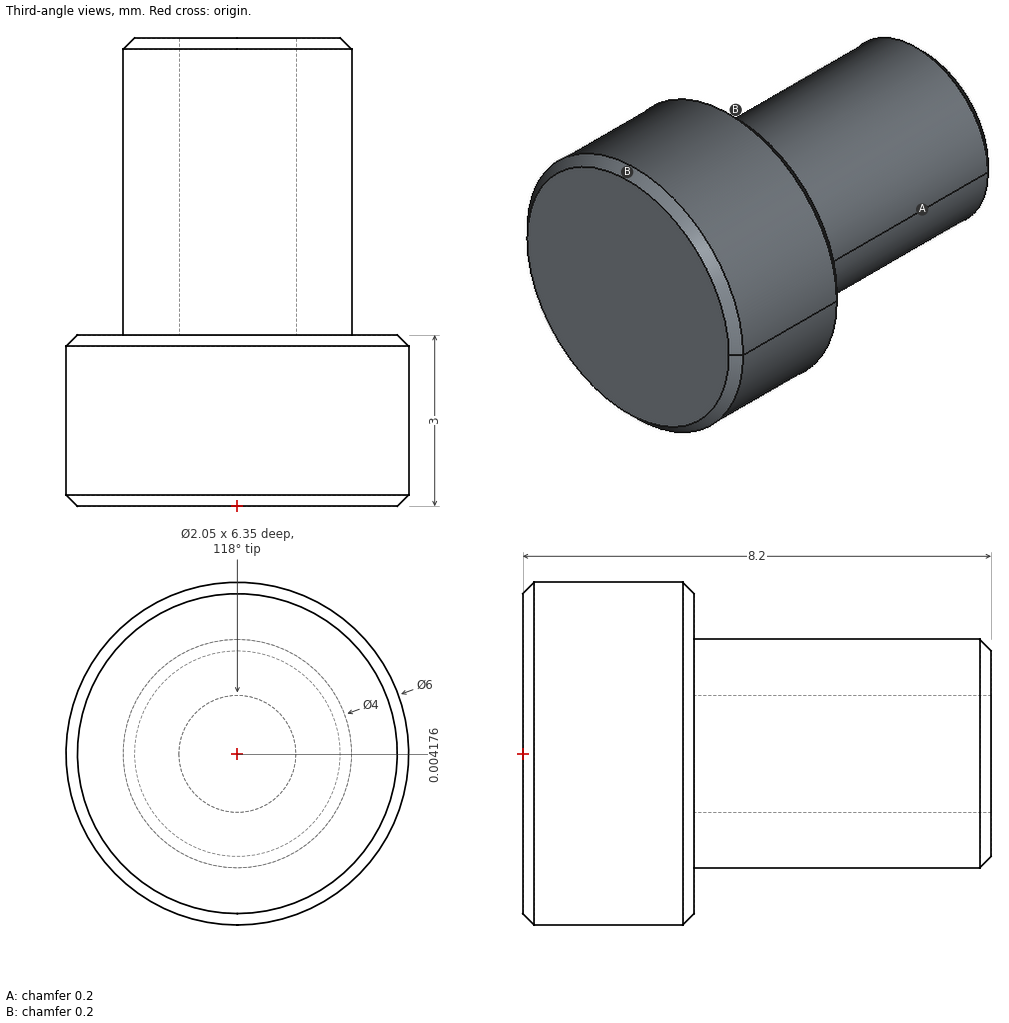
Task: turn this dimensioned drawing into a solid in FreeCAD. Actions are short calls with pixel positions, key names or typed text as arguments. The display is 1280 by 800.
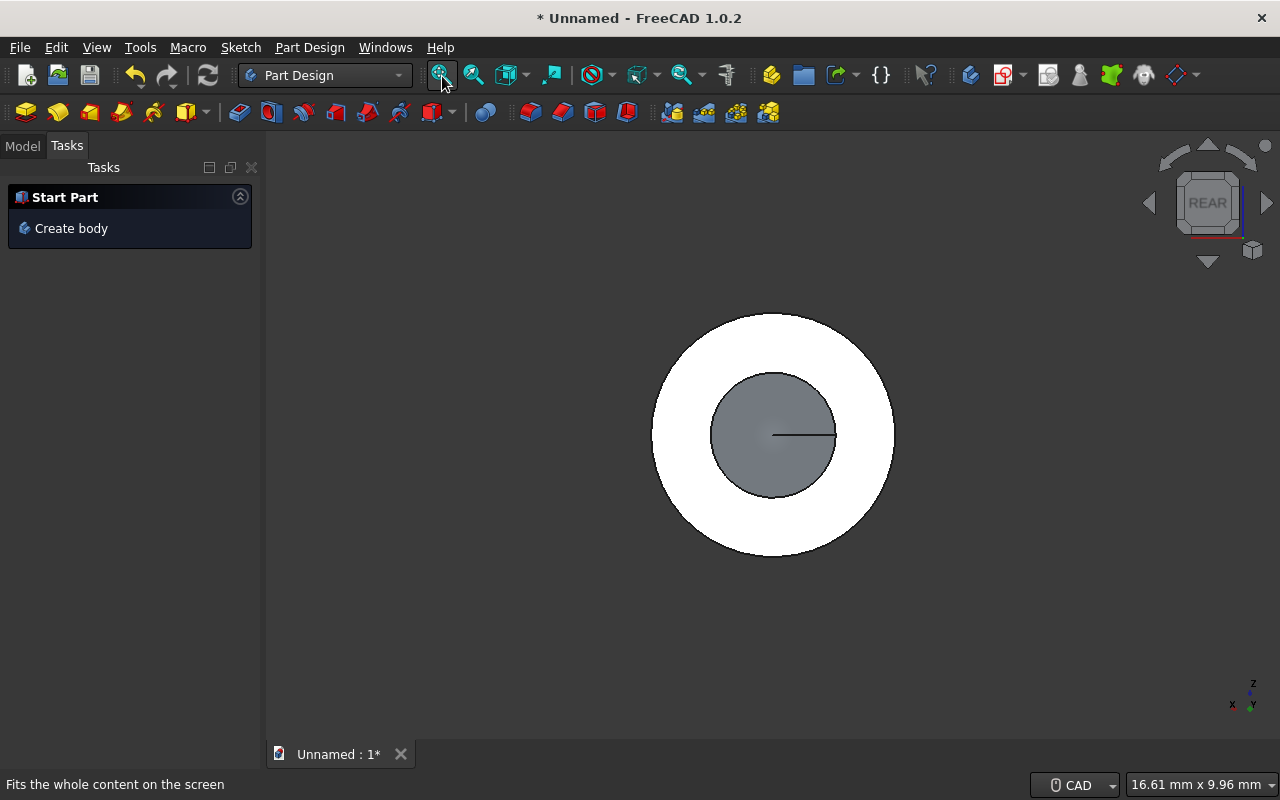
click(1004, 76)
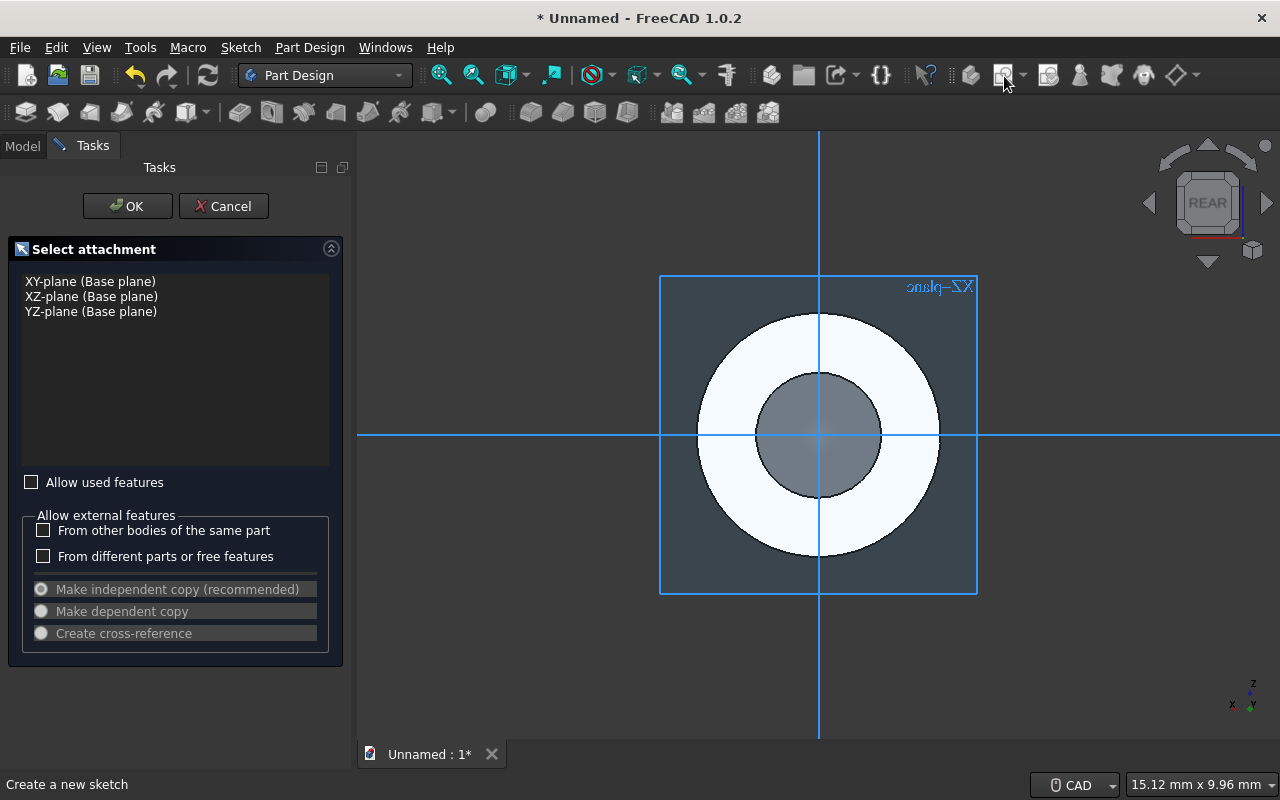
click(82, 296)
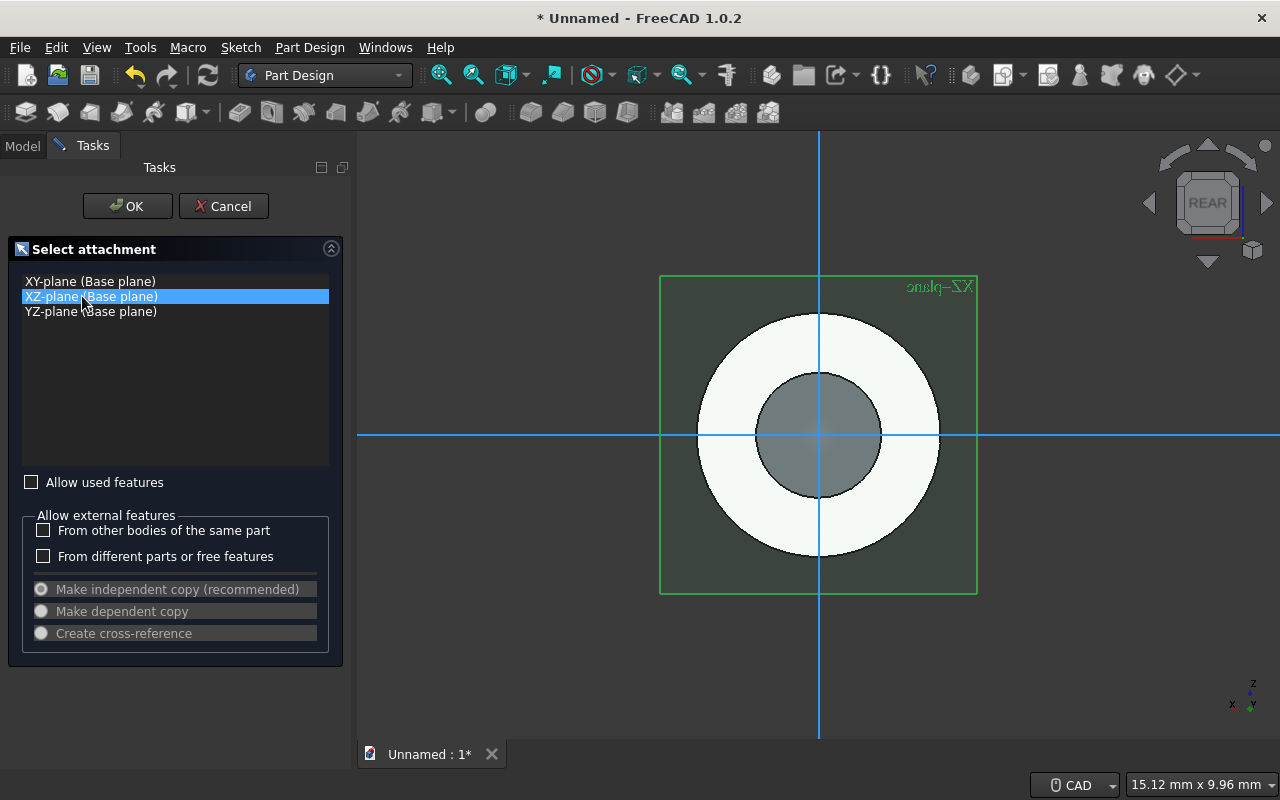
click(128, 206)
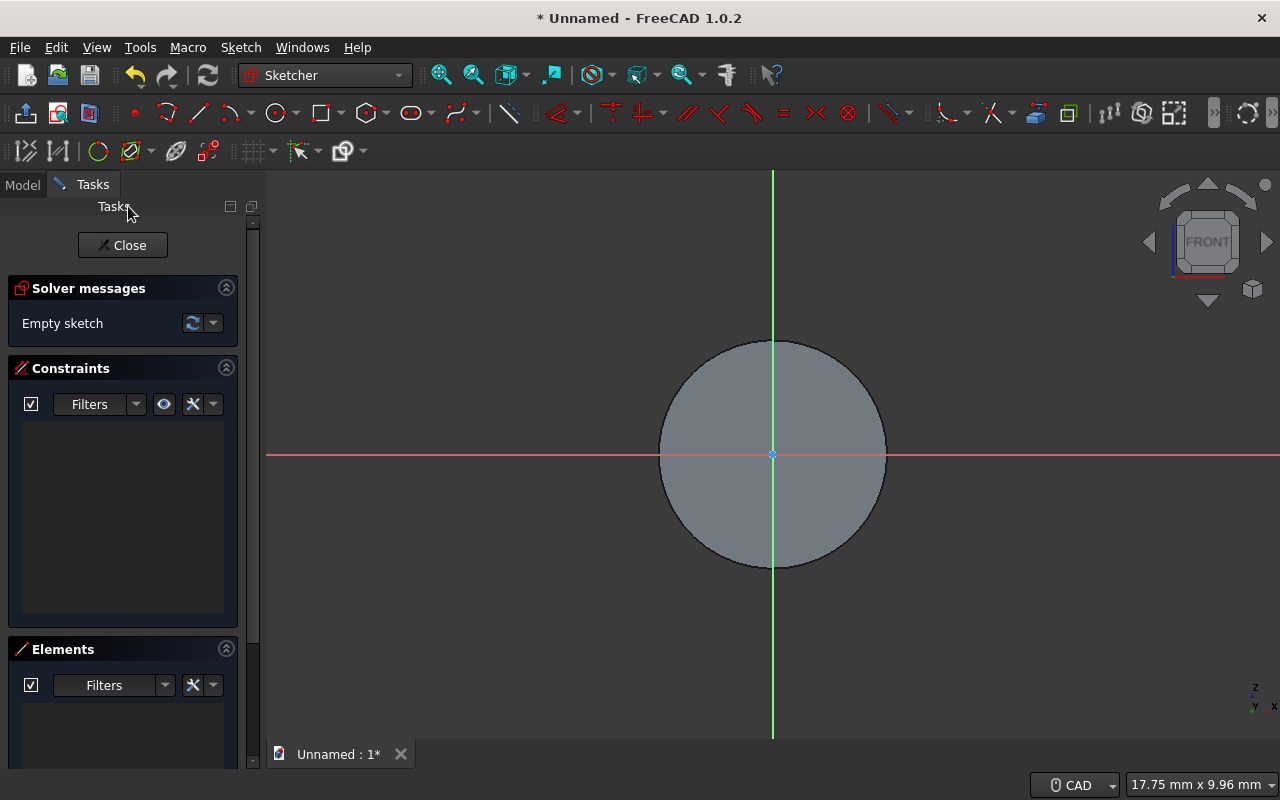
click(276, 114)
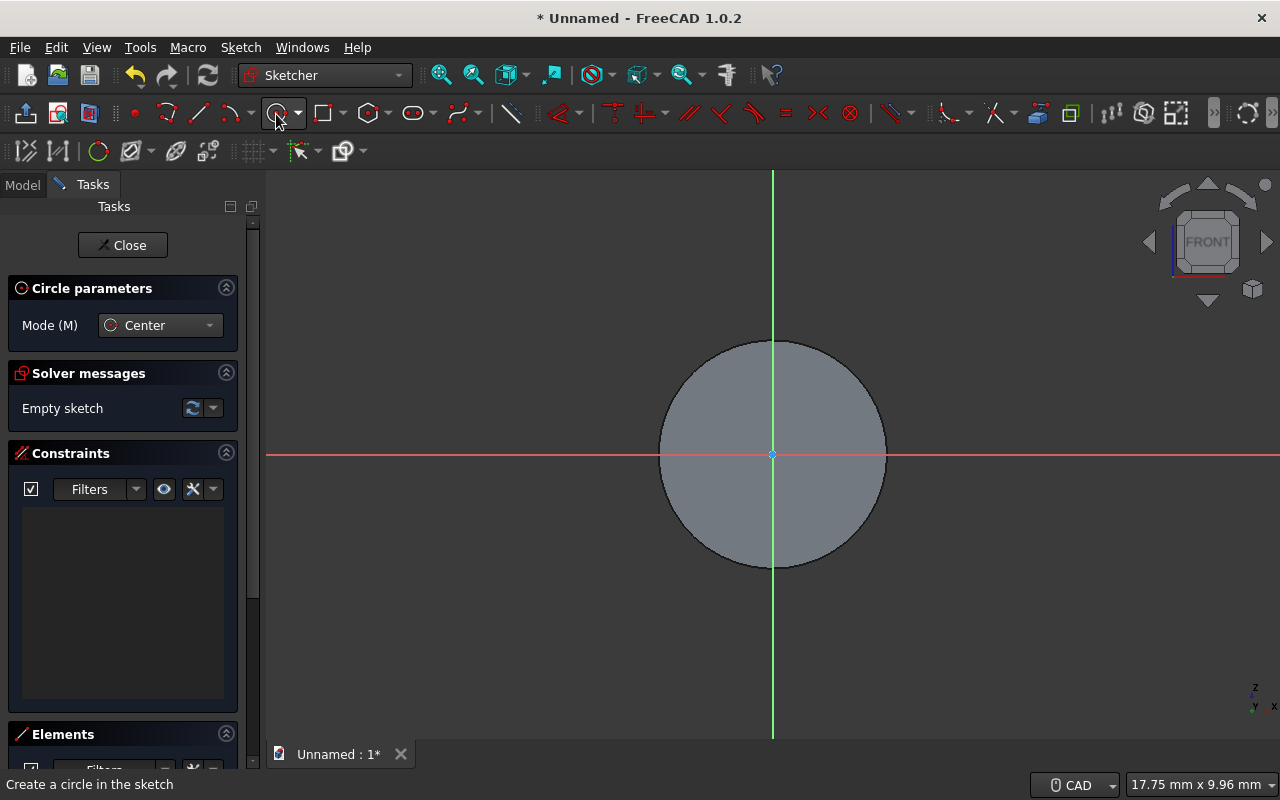
click(773, 455)
click(894, 333)
key(Escape)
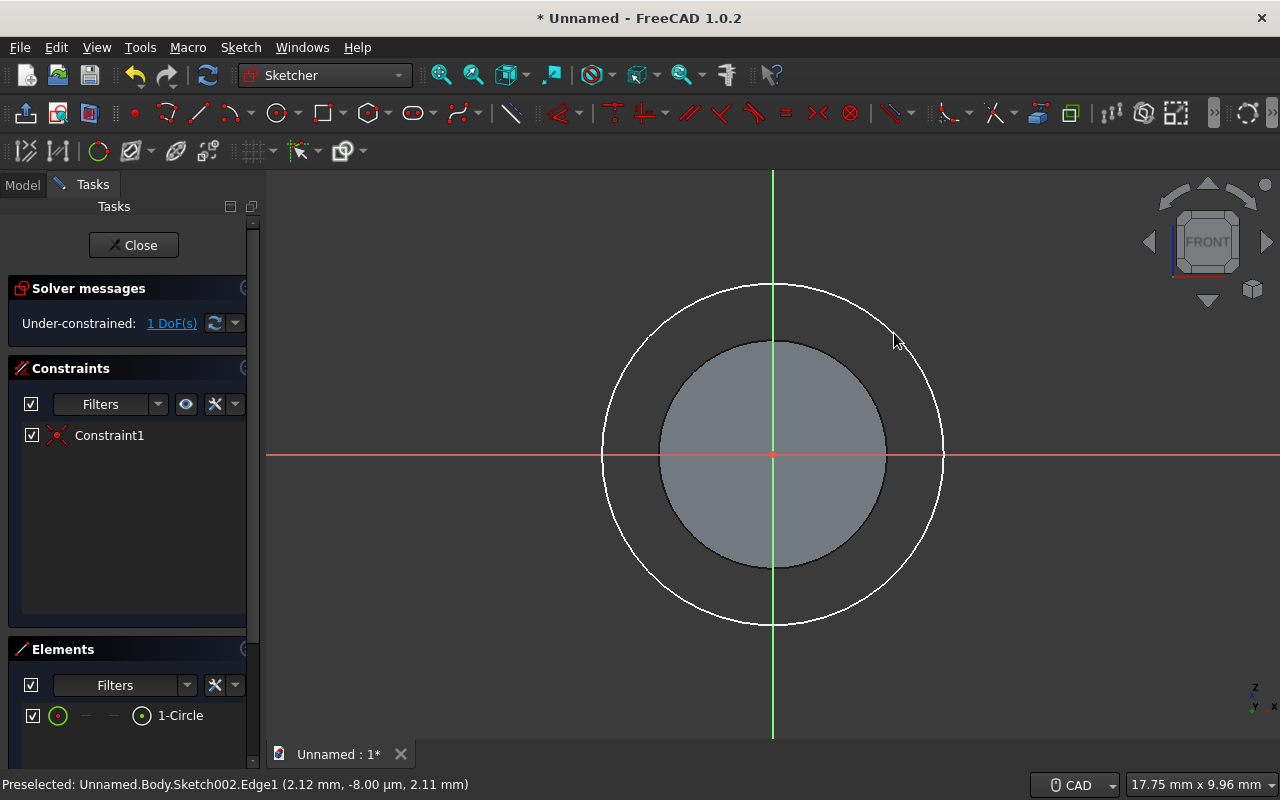
click(558, 114)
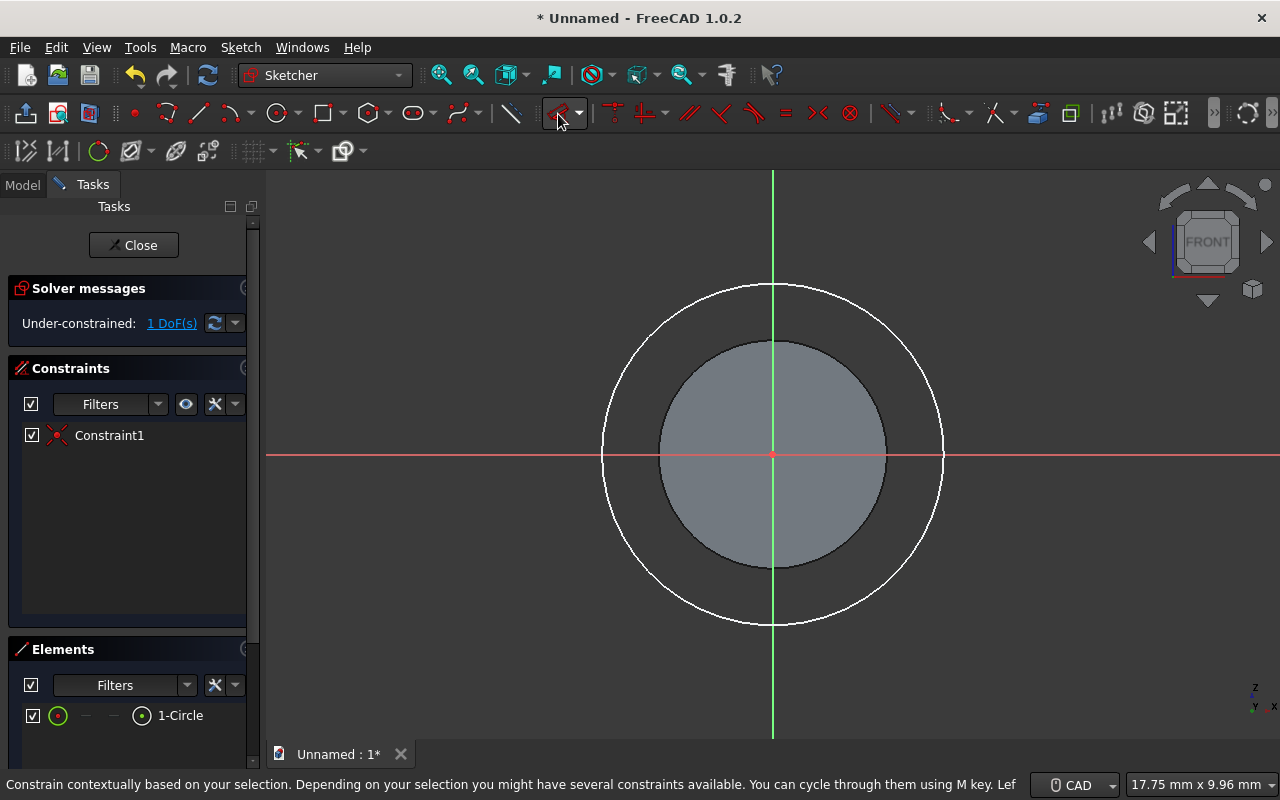
click(893, 333)
click(916, 310)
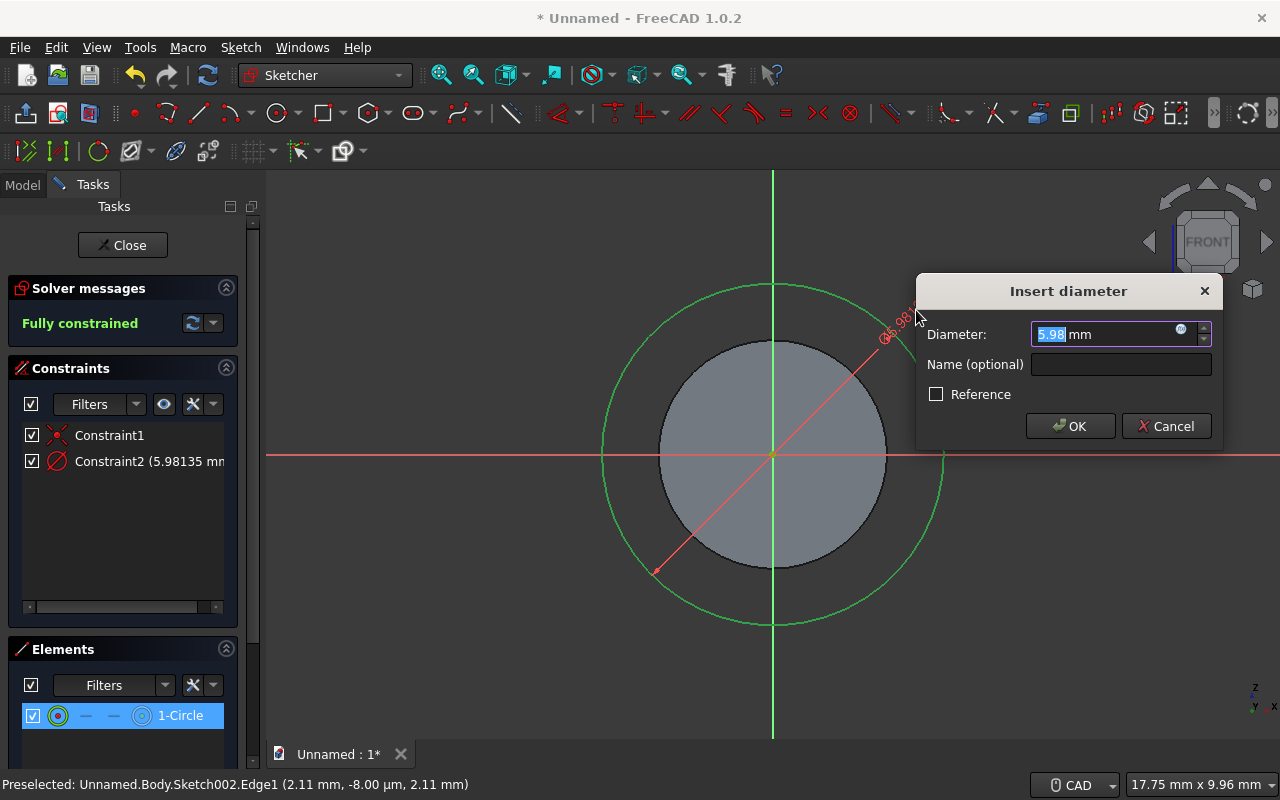
text(6)
key(Return)
key(Escape)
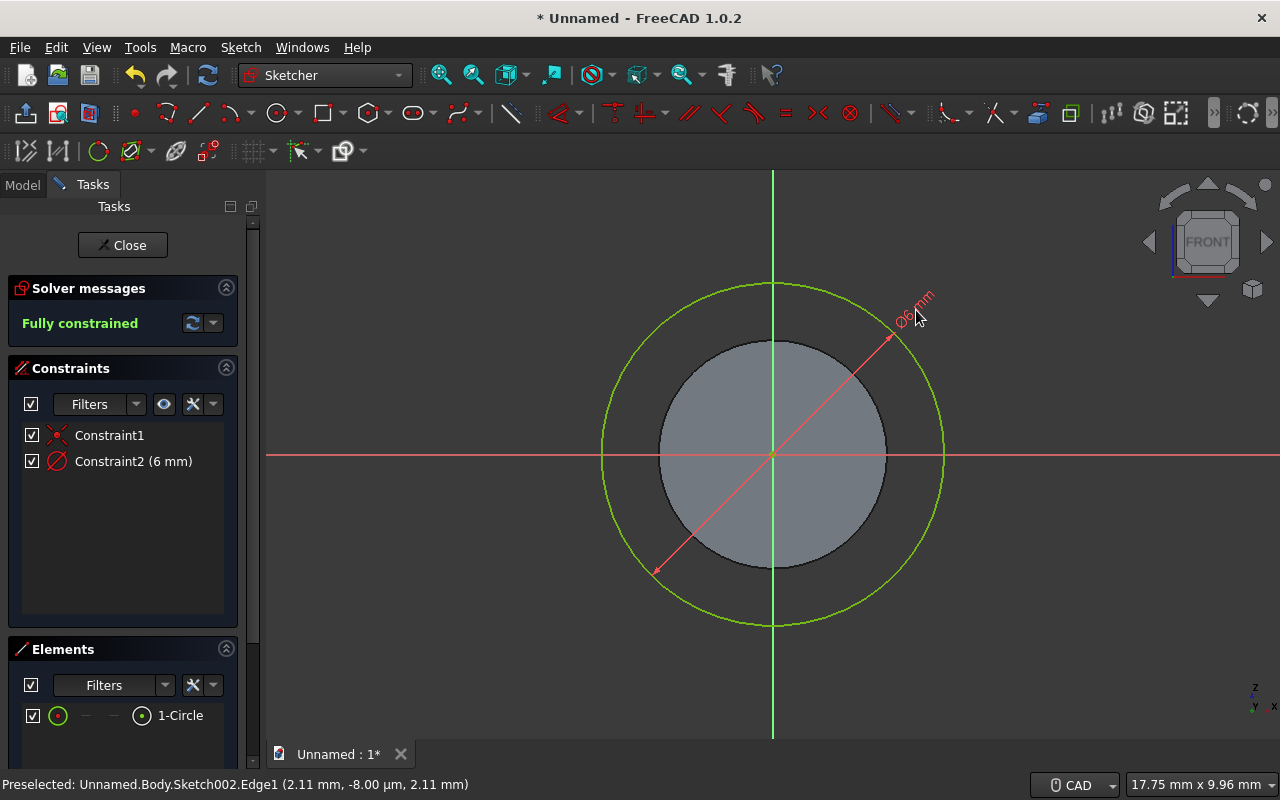
click(123, 245)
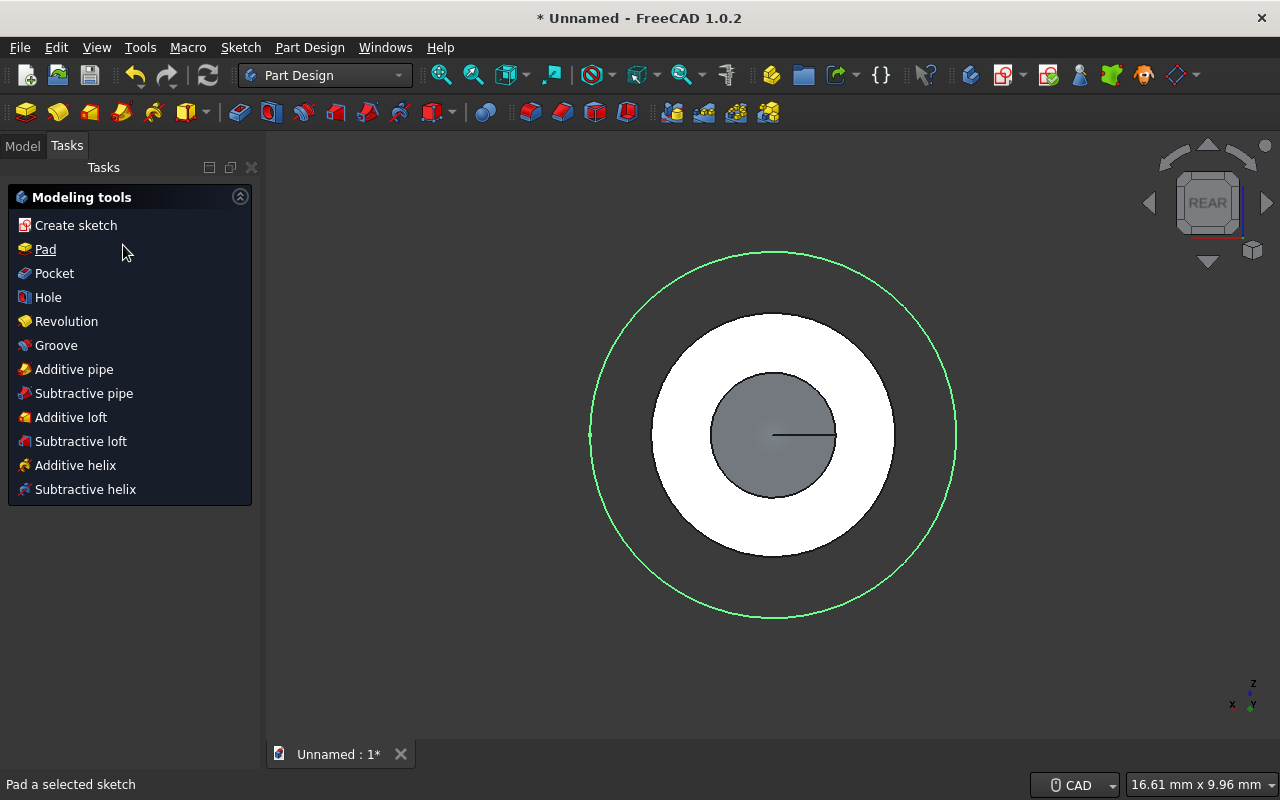
click(26, 112)